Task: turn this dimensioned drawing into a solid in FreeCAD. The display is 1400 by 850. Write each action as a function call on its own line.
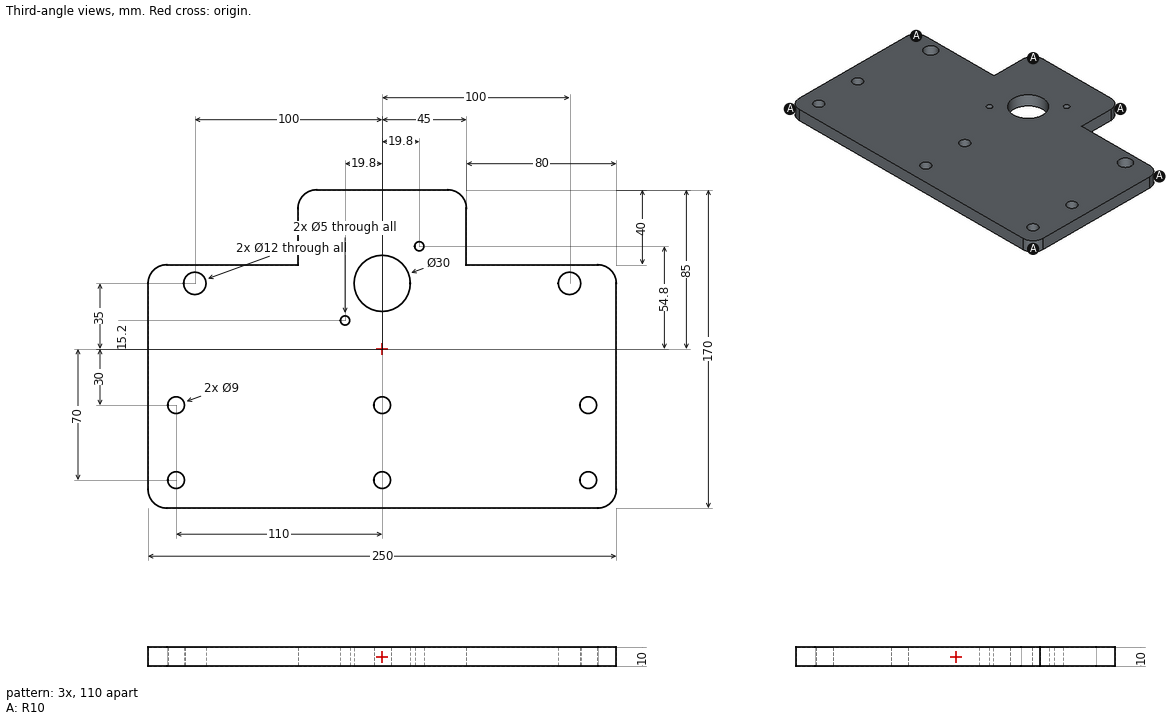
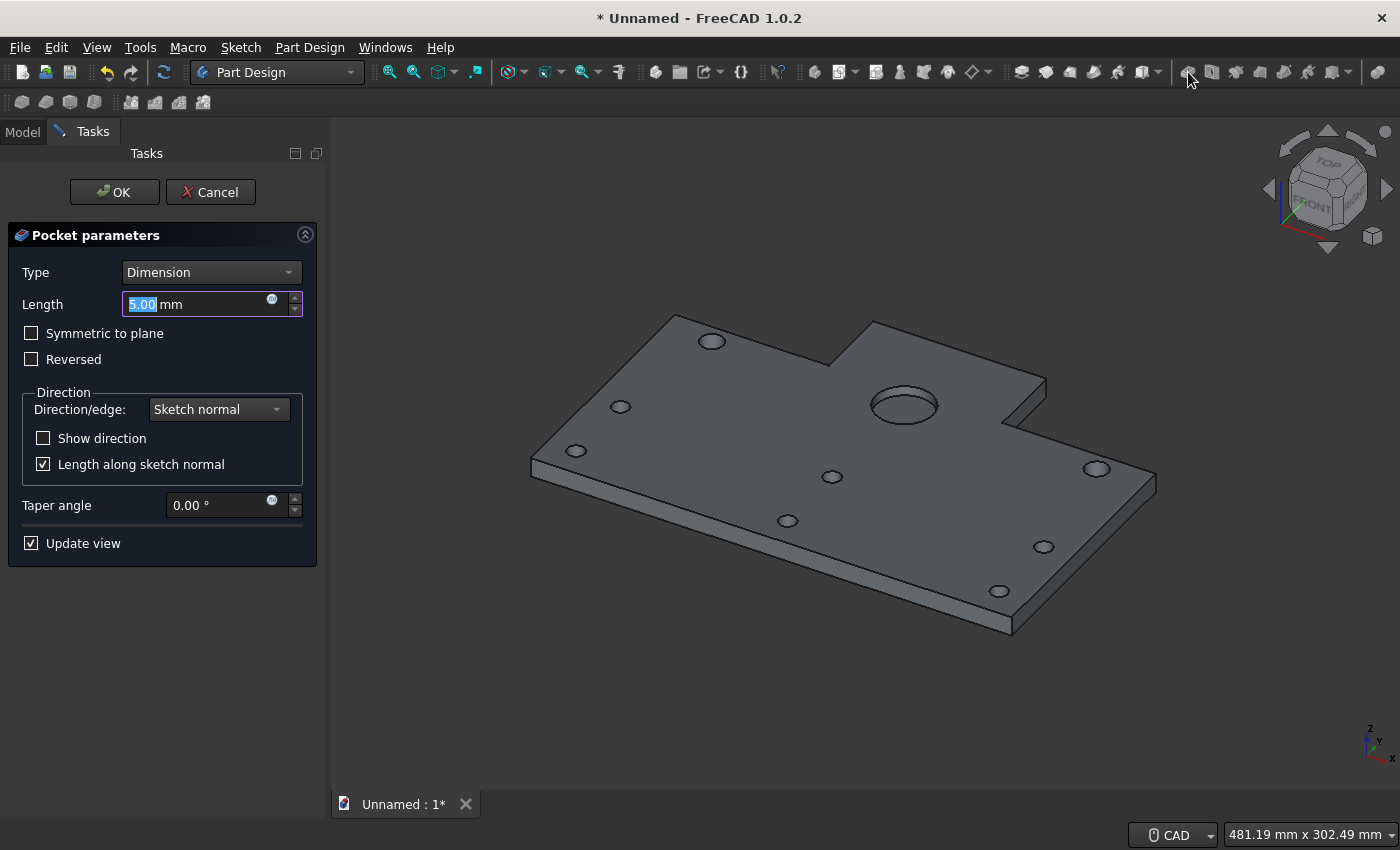
text(10)
key(Tab)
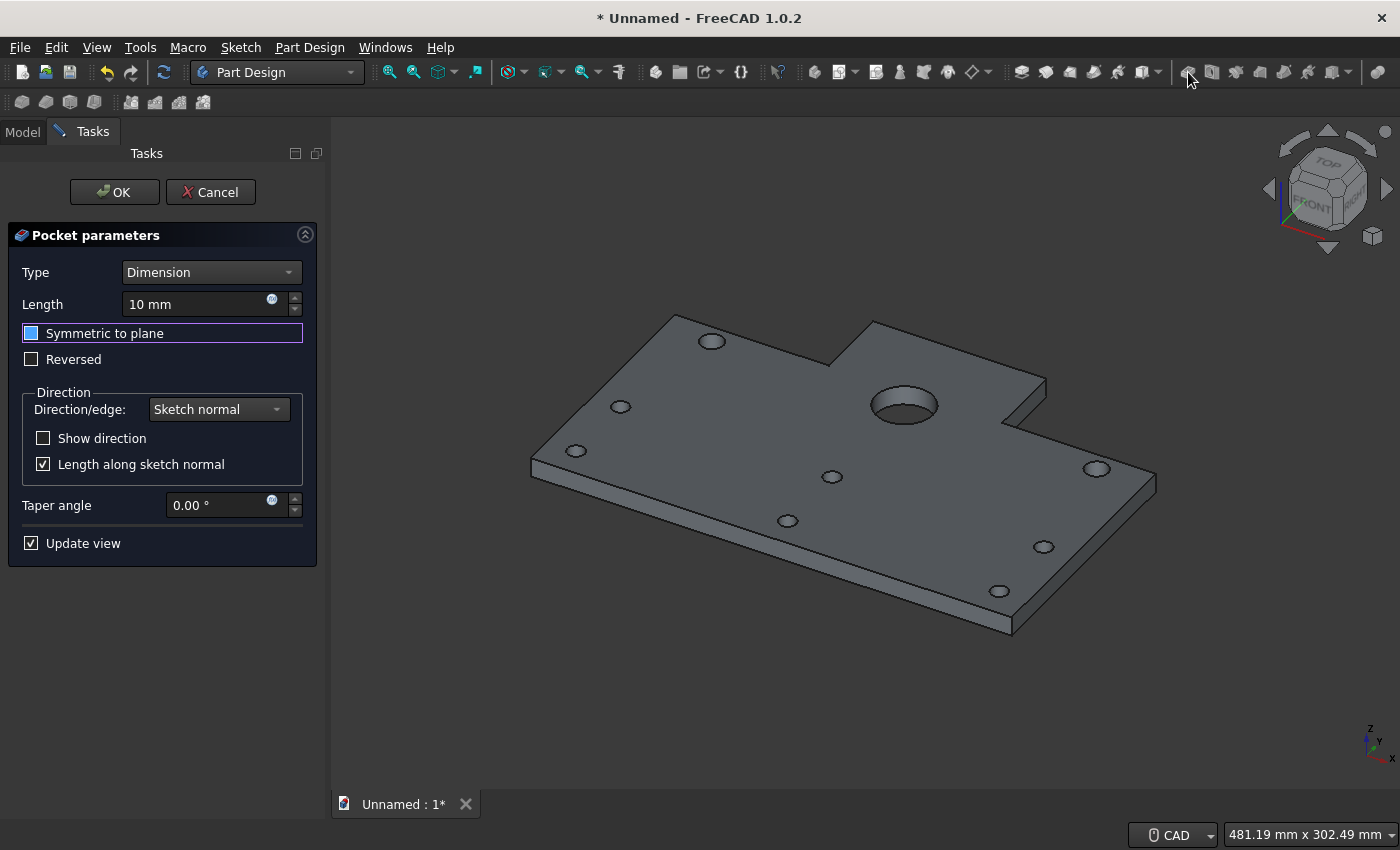
click(115, 192)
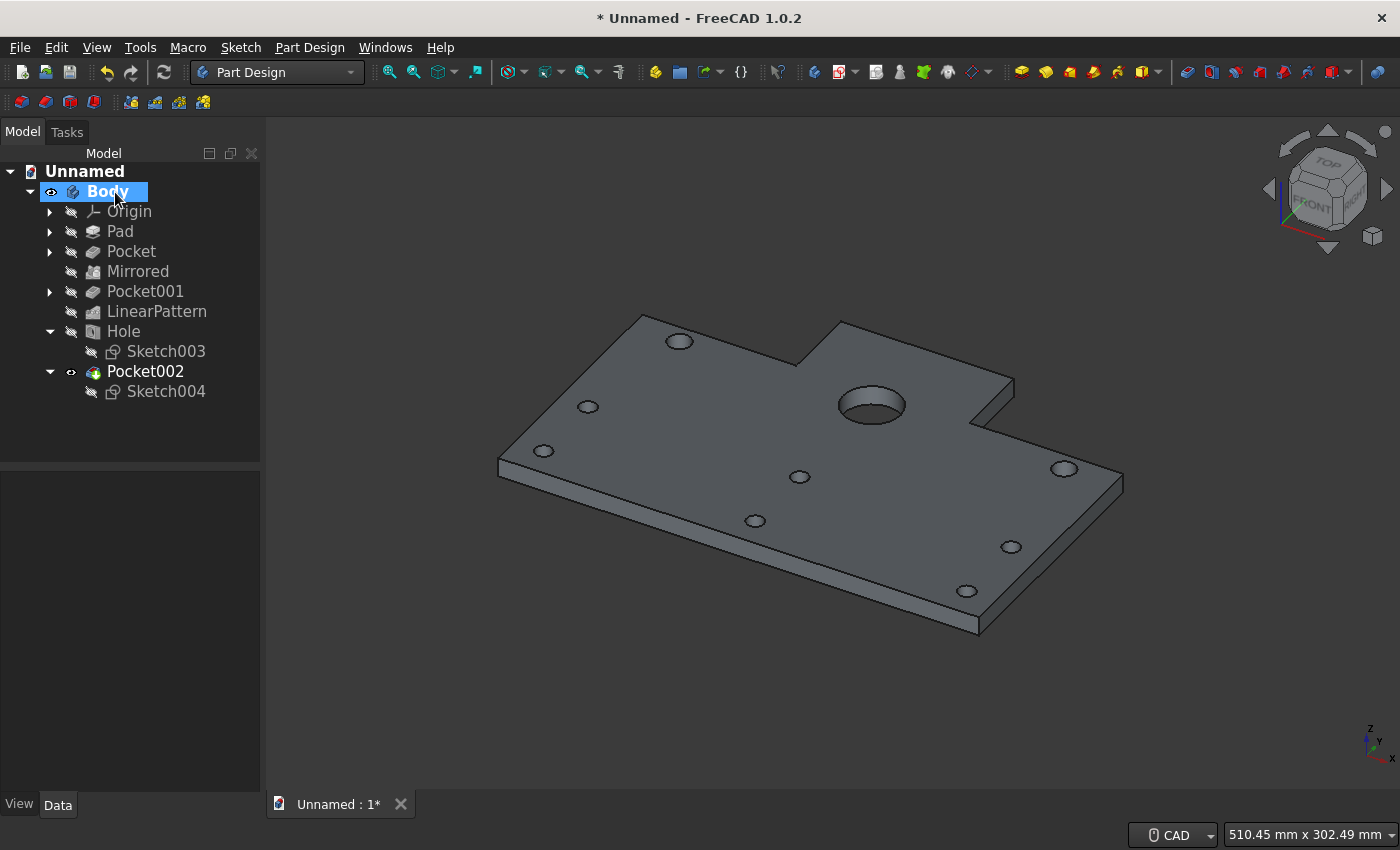
click(970, 488)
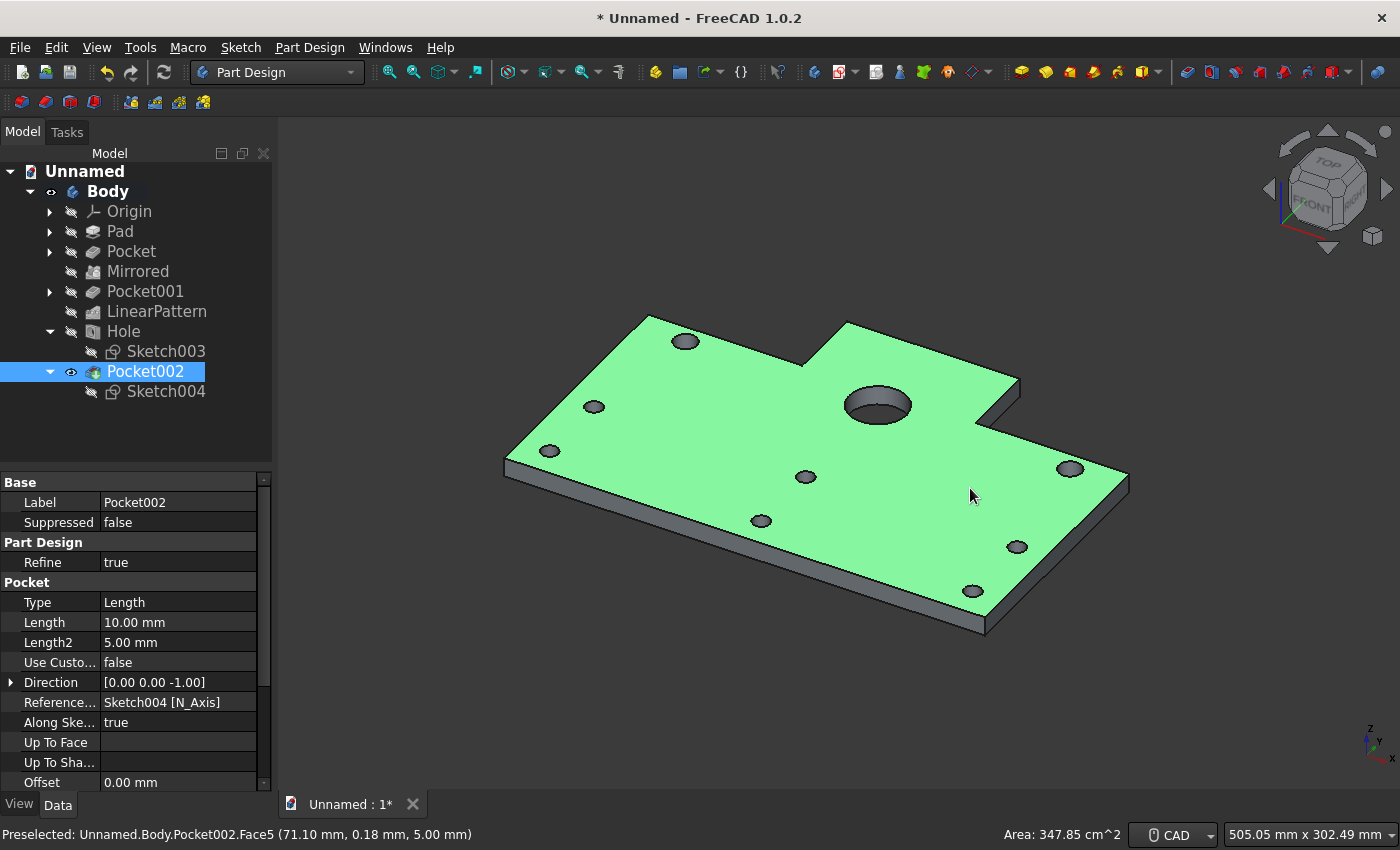
click(840, 72)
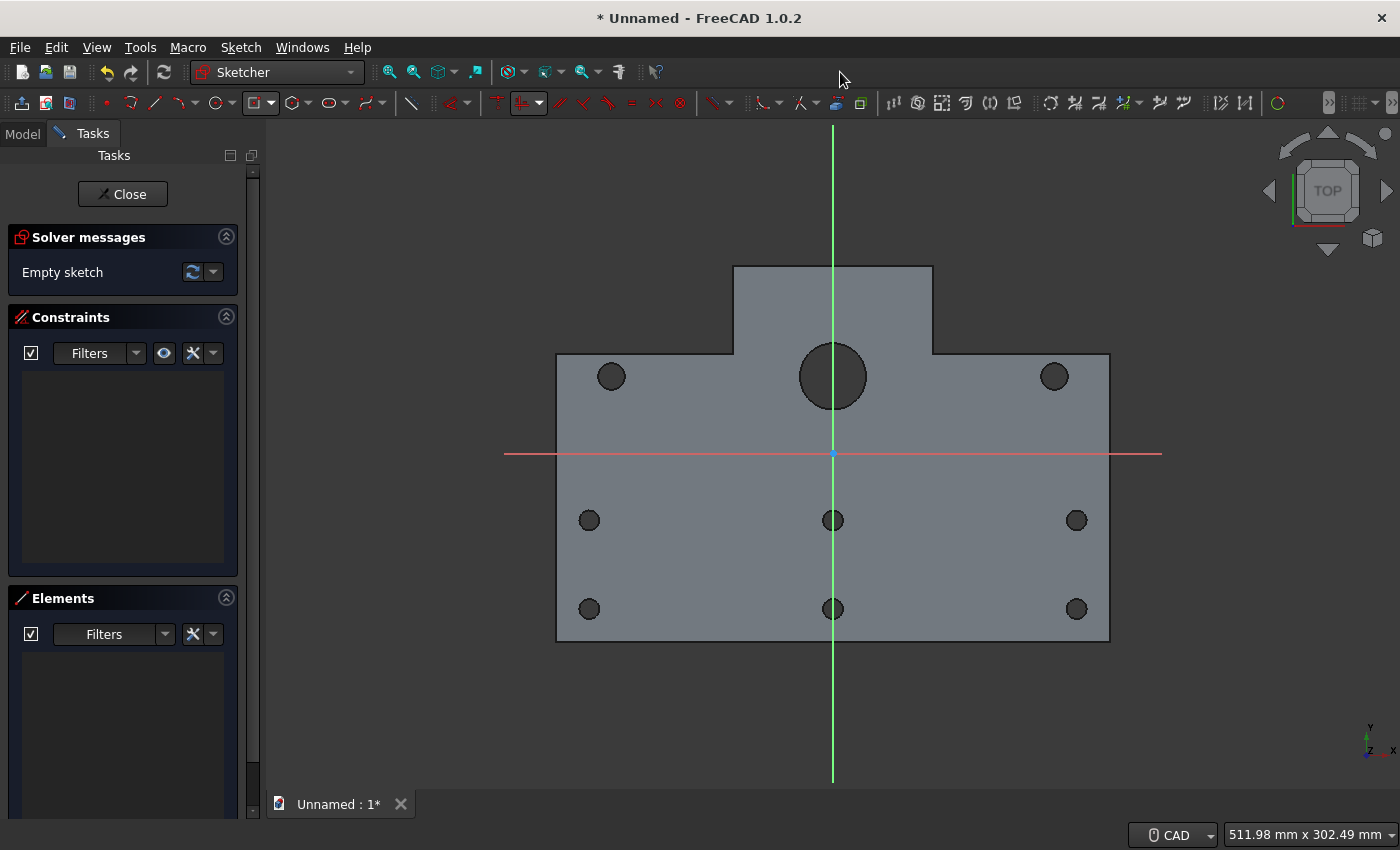
scroll(863, 363, up, 6)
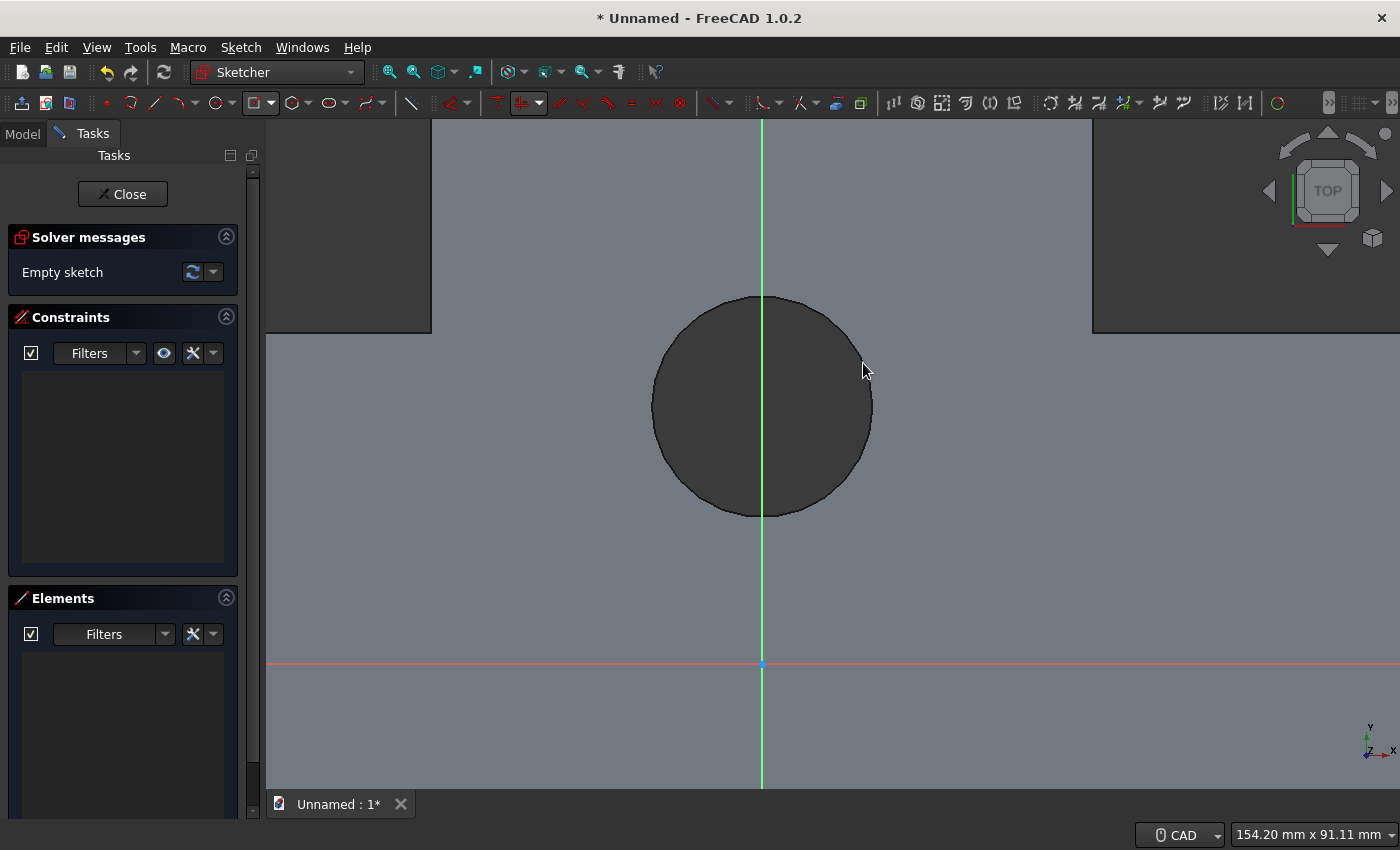
click(216, 104)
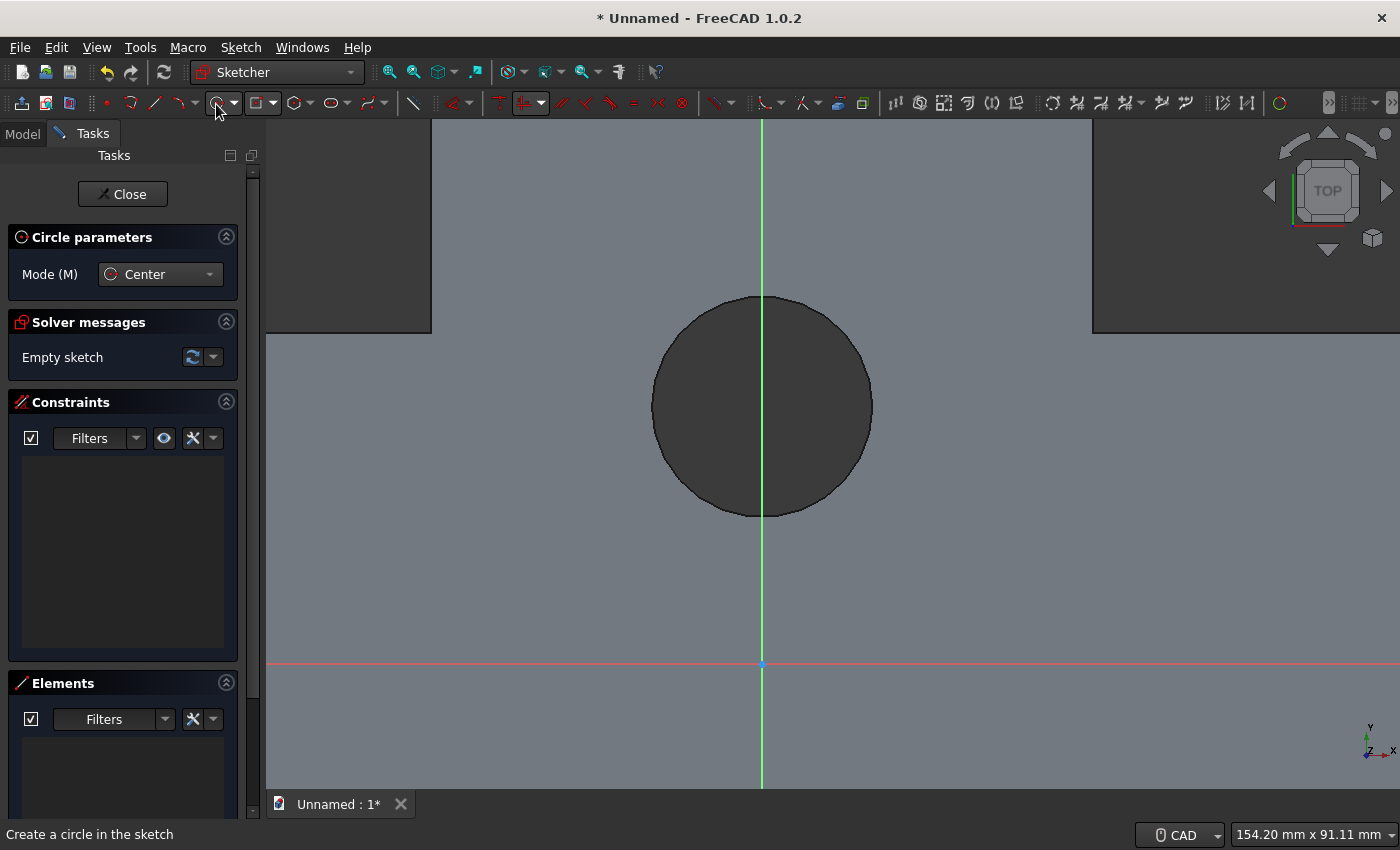
scroll(617, 553, up, 2)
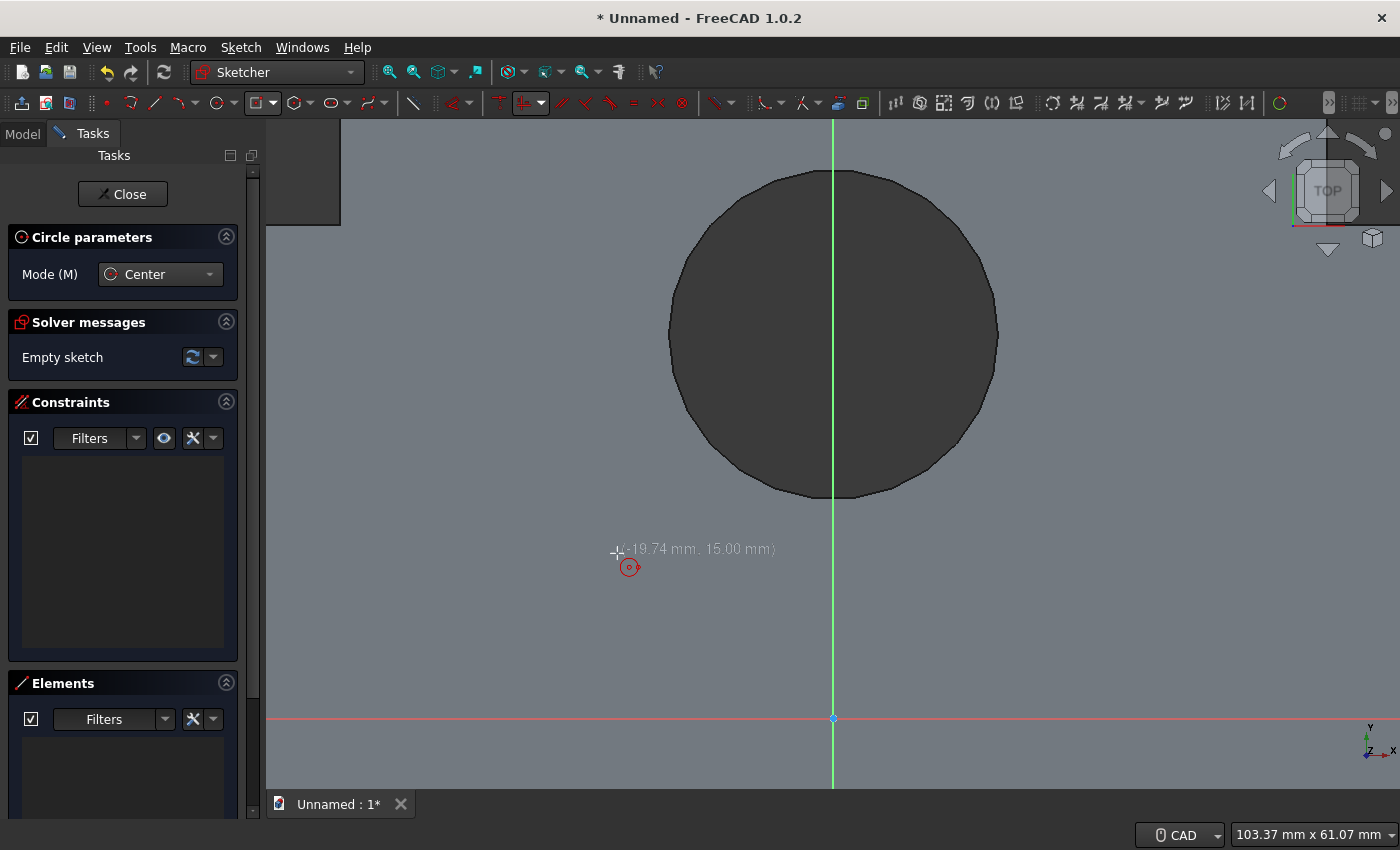
click(616, 552)
move(636, 533)